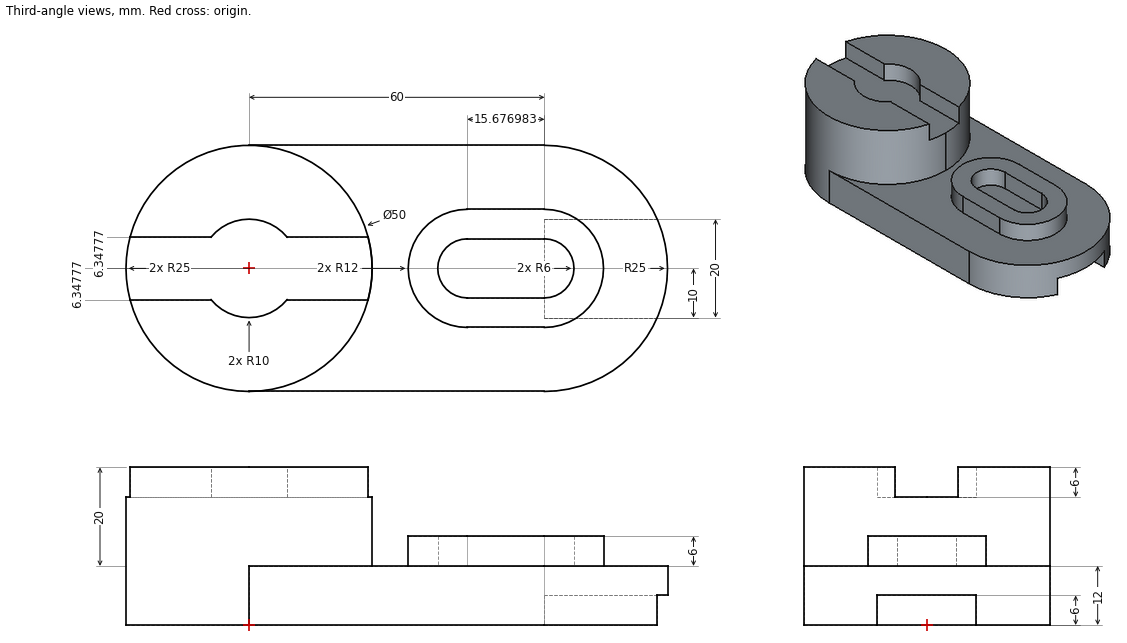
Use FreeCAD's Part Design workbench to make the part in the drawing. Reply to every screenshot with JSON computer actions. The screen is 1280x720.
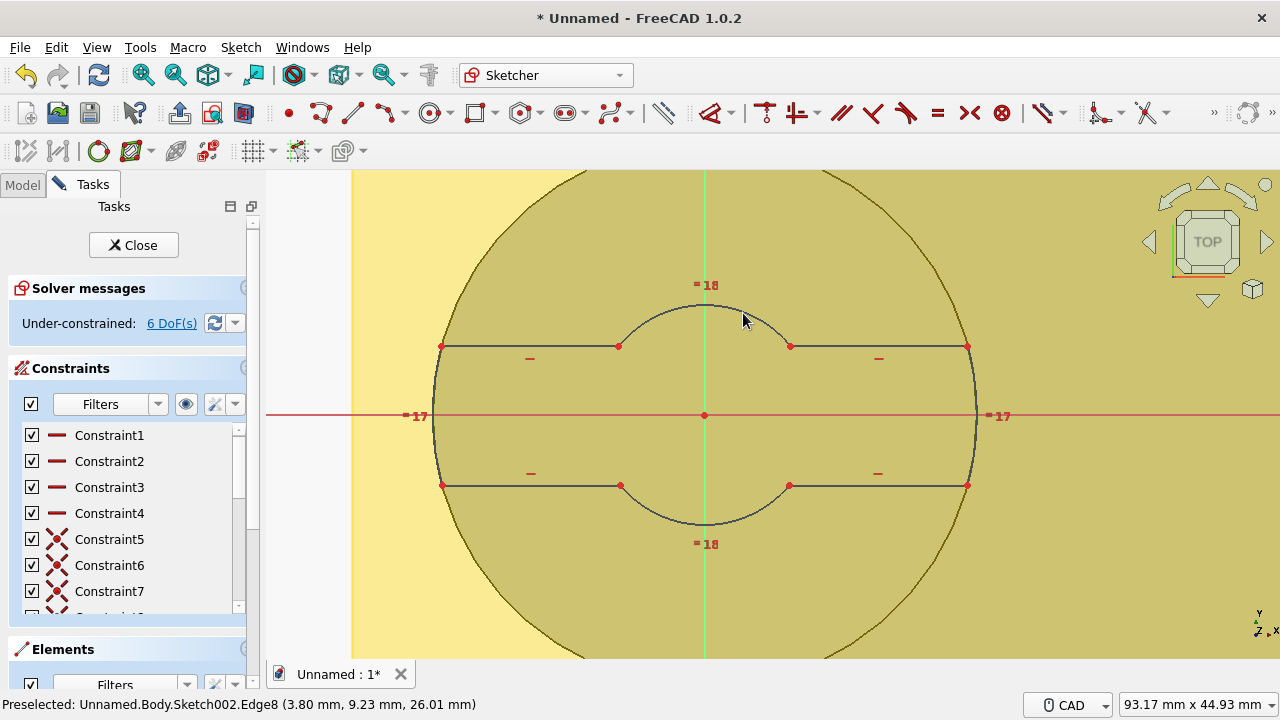
{"action": "left_click", "coordinate": [710, 114]}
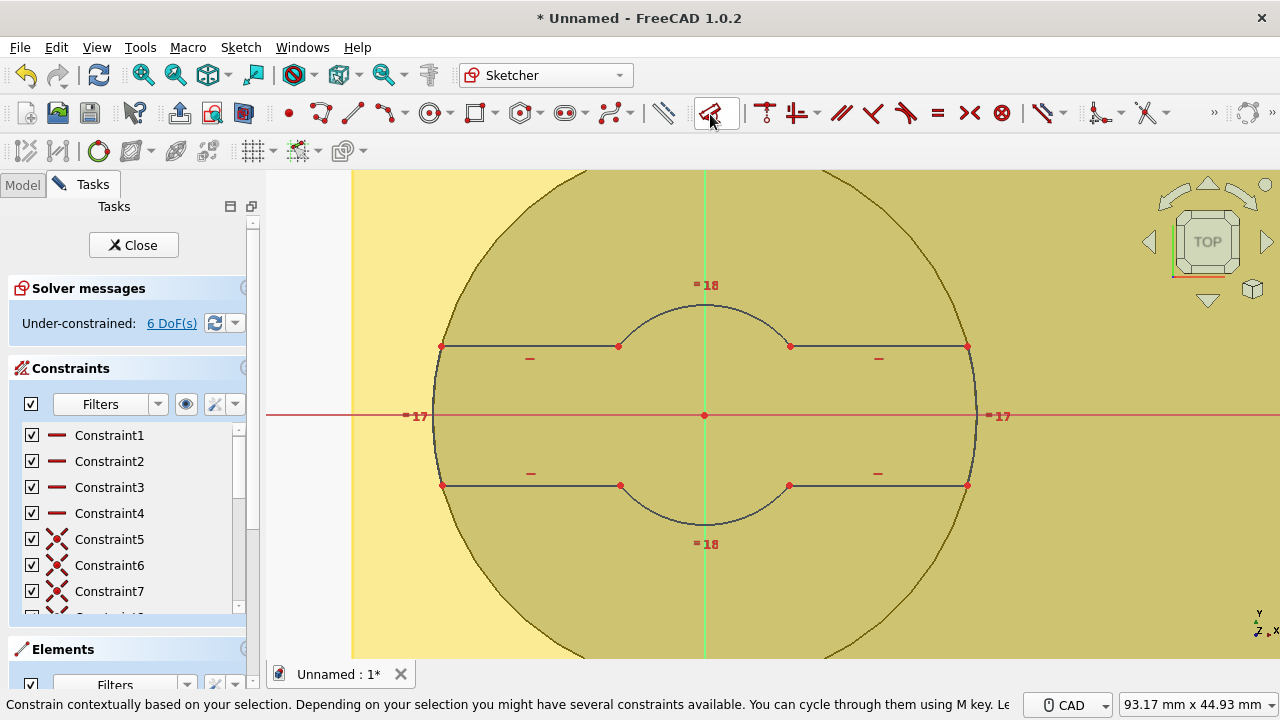
{"action": "left_click", "coordinate": [434, 388]}
{"action": "left_click", "coordinate": [402, 385]}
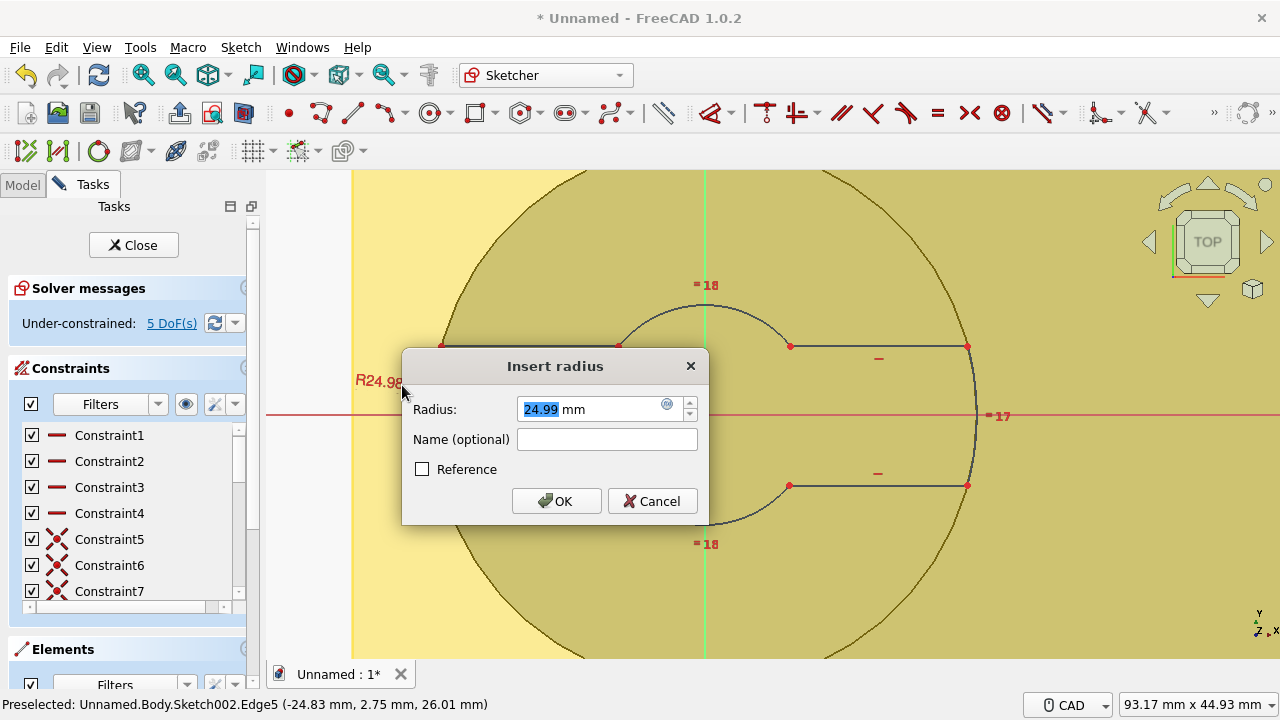
{"action": "type", "text": "25"}
{"action": "key", "text": "Return"}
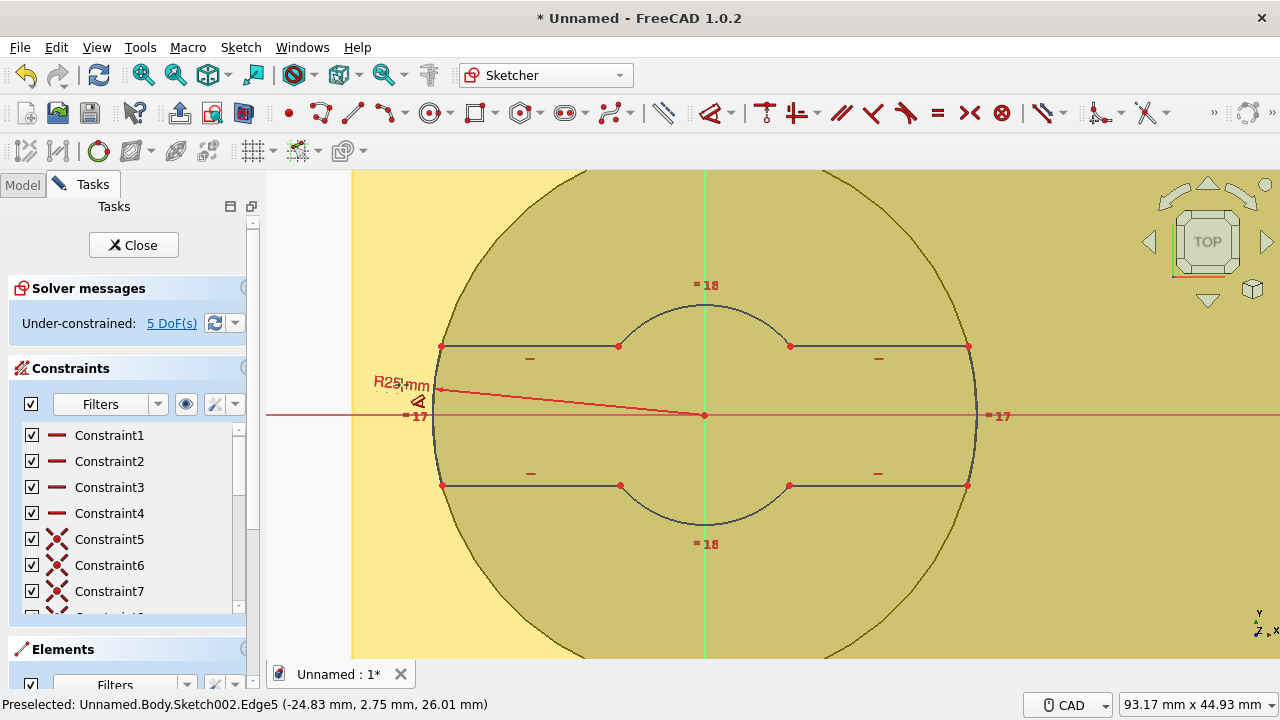
{"action": "left_click", "coordinate": [667, 518]}
{"action": "left_click", "coordinate": [656, 548]}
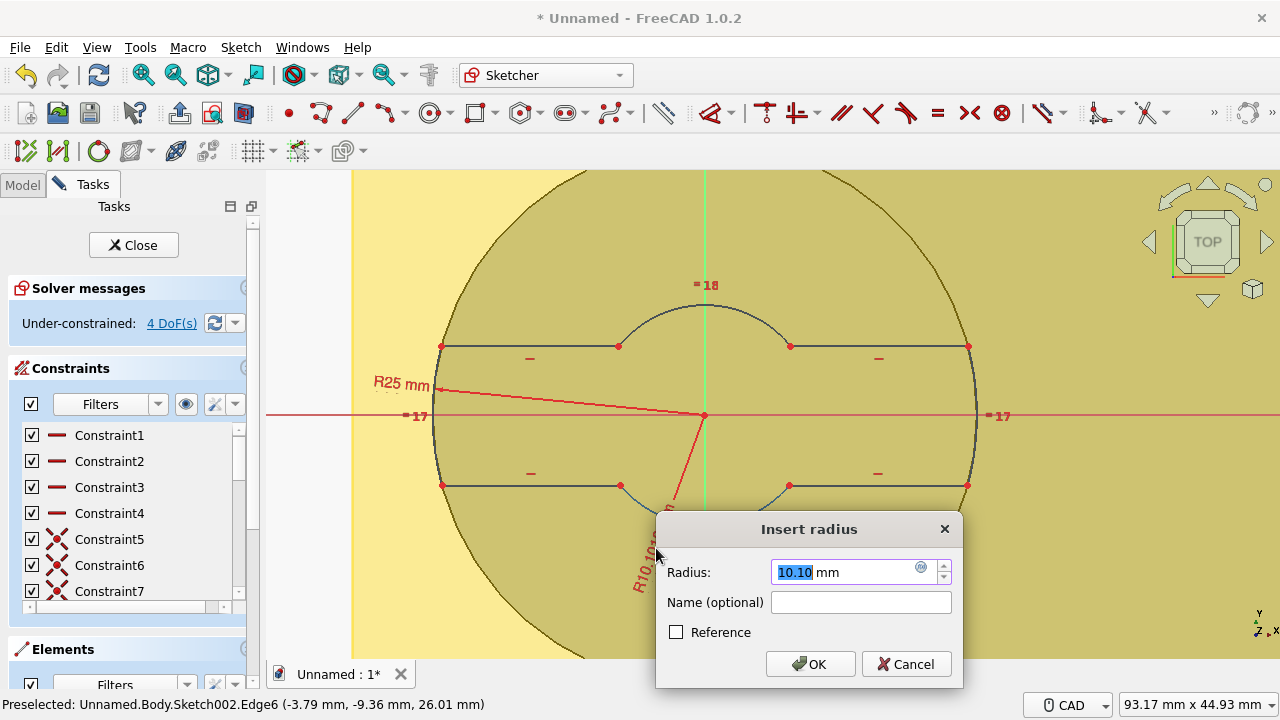
{"action": "type", "text": "10"}
{"action": "key", "text": "Return"}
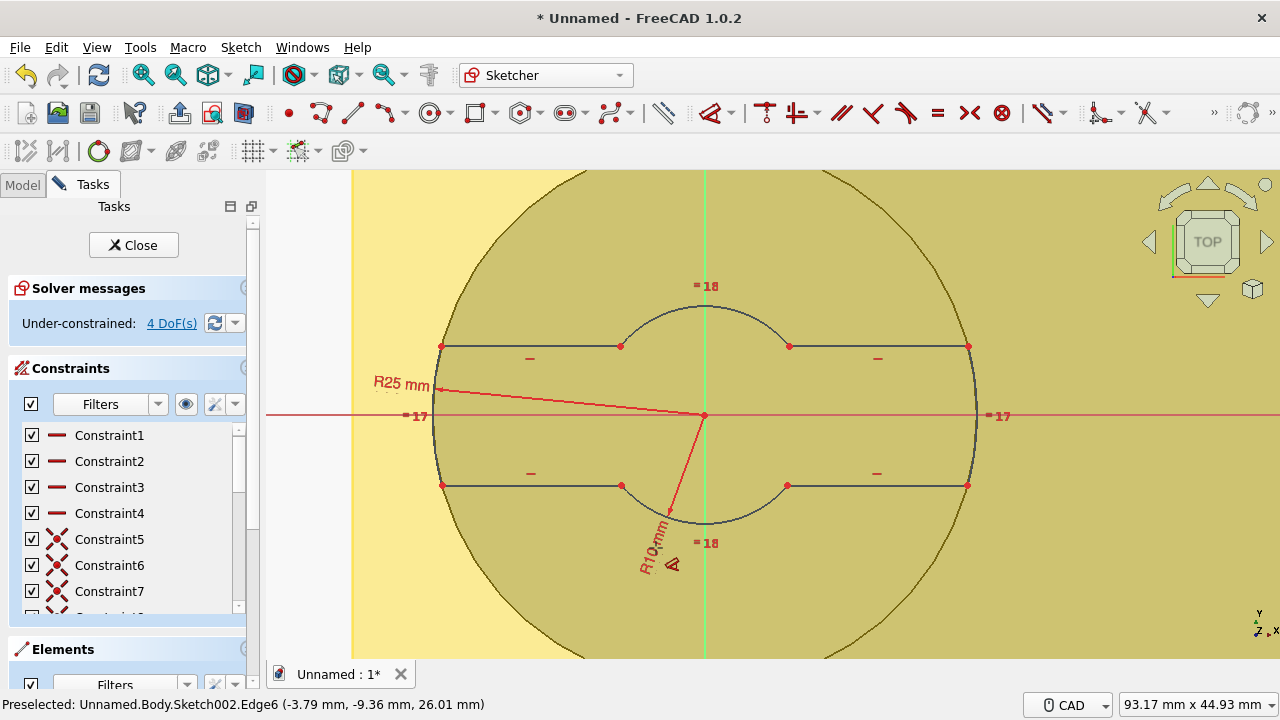
{"action": "left_click", "coordinate": [620, 346]}
{"action": "left_click", "coordinate": [586, 381]}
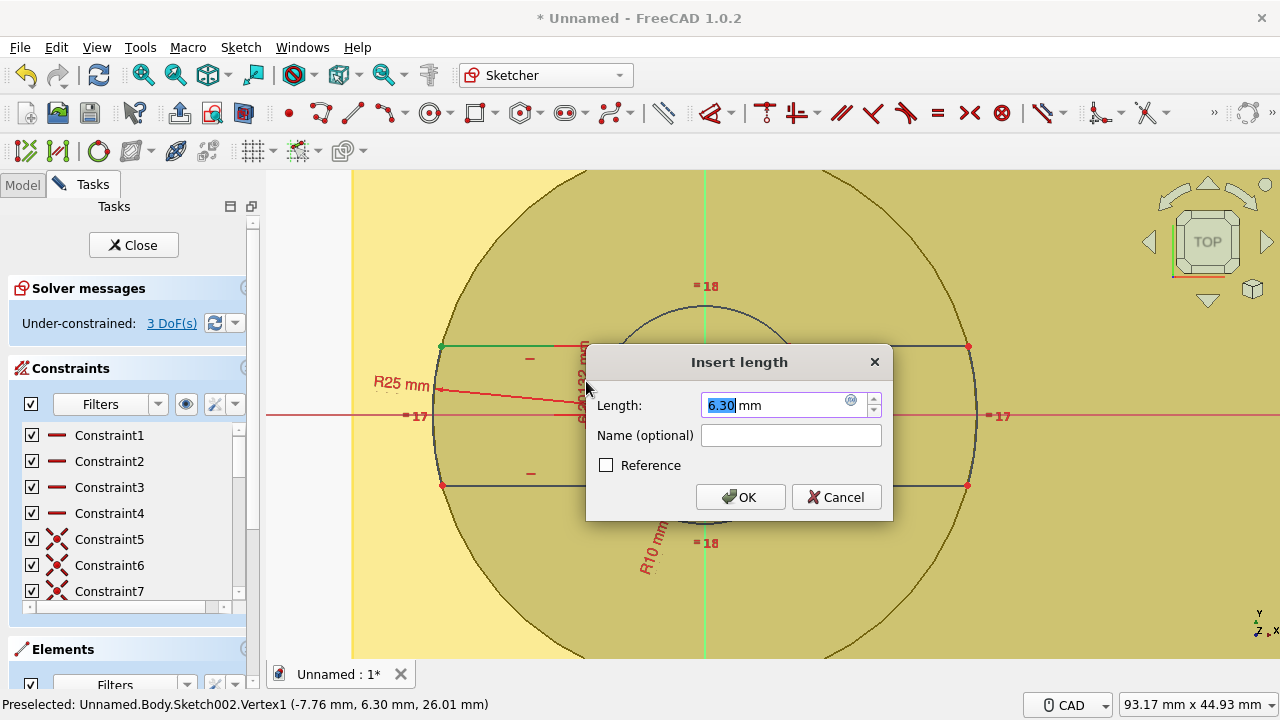
{"action": "type", "text": "6.34777"}
{"action": "key", "text": "Return"}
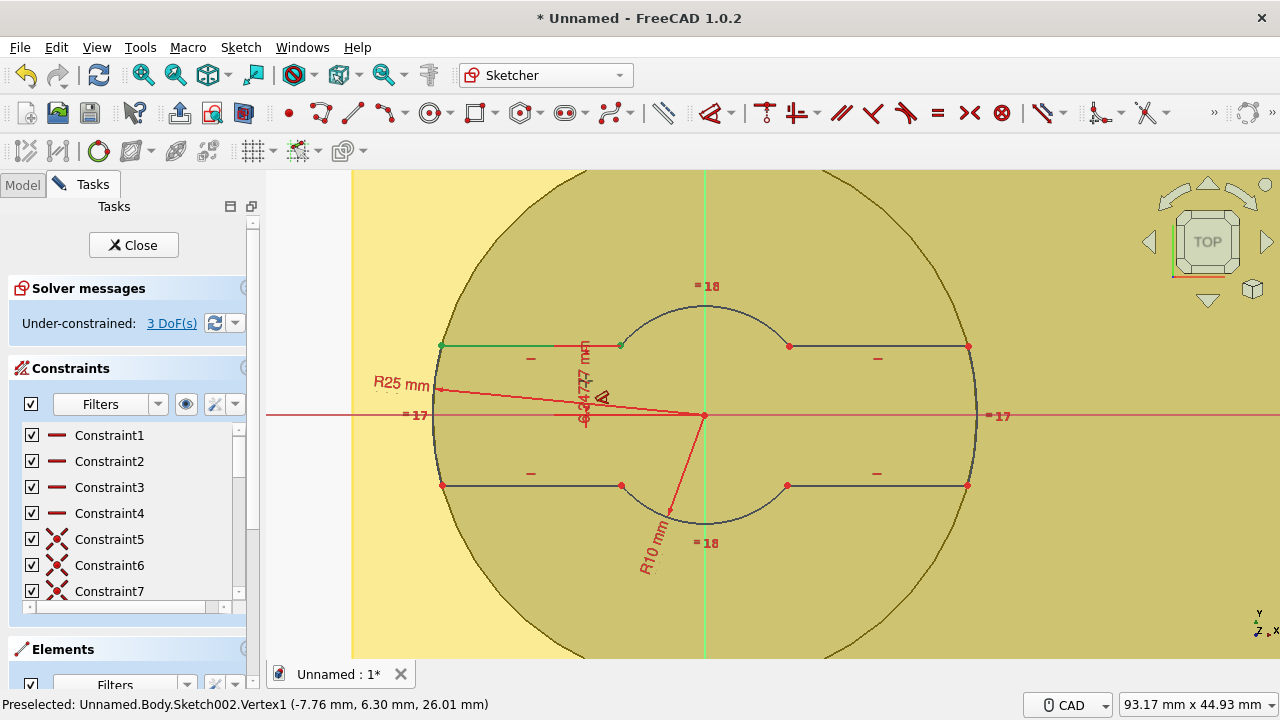
{"action": "left_click", "coordinate": [442, 486]}
{"action": "left_click", "coordinate": [408, 450]}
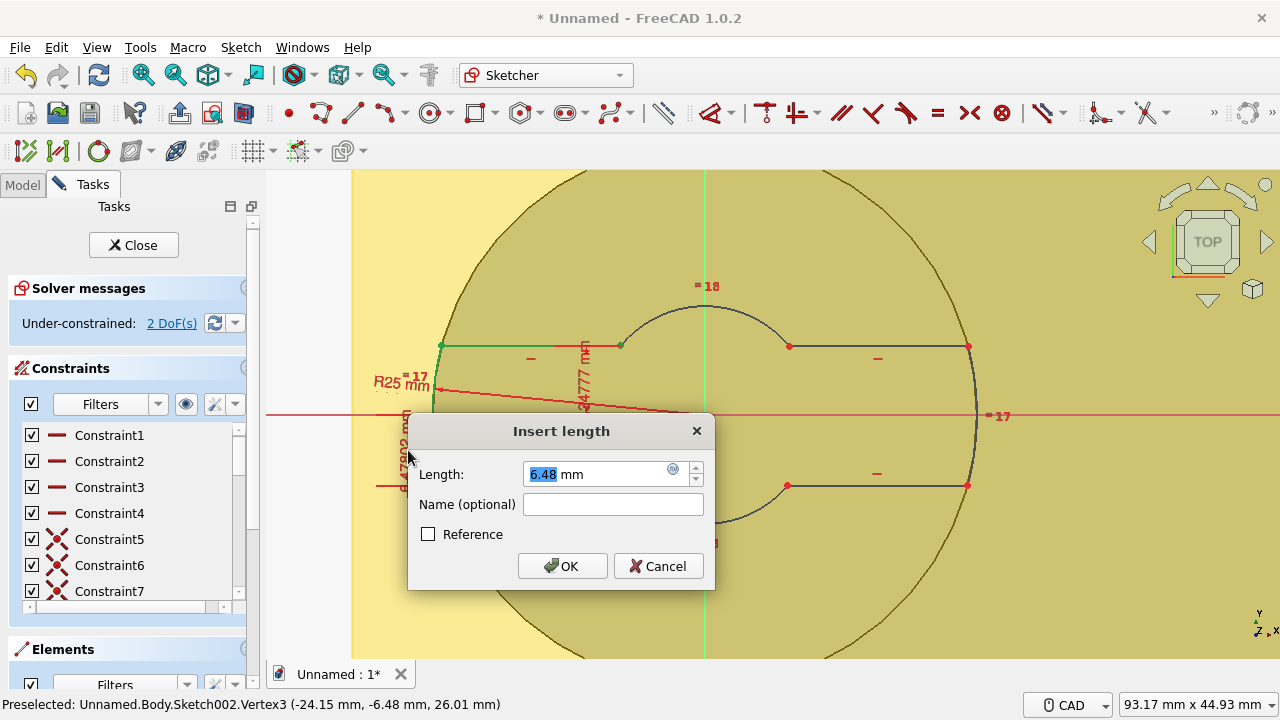
{"action": "type", "text": "6.34777"}
{"action": "key", "text": "Return"}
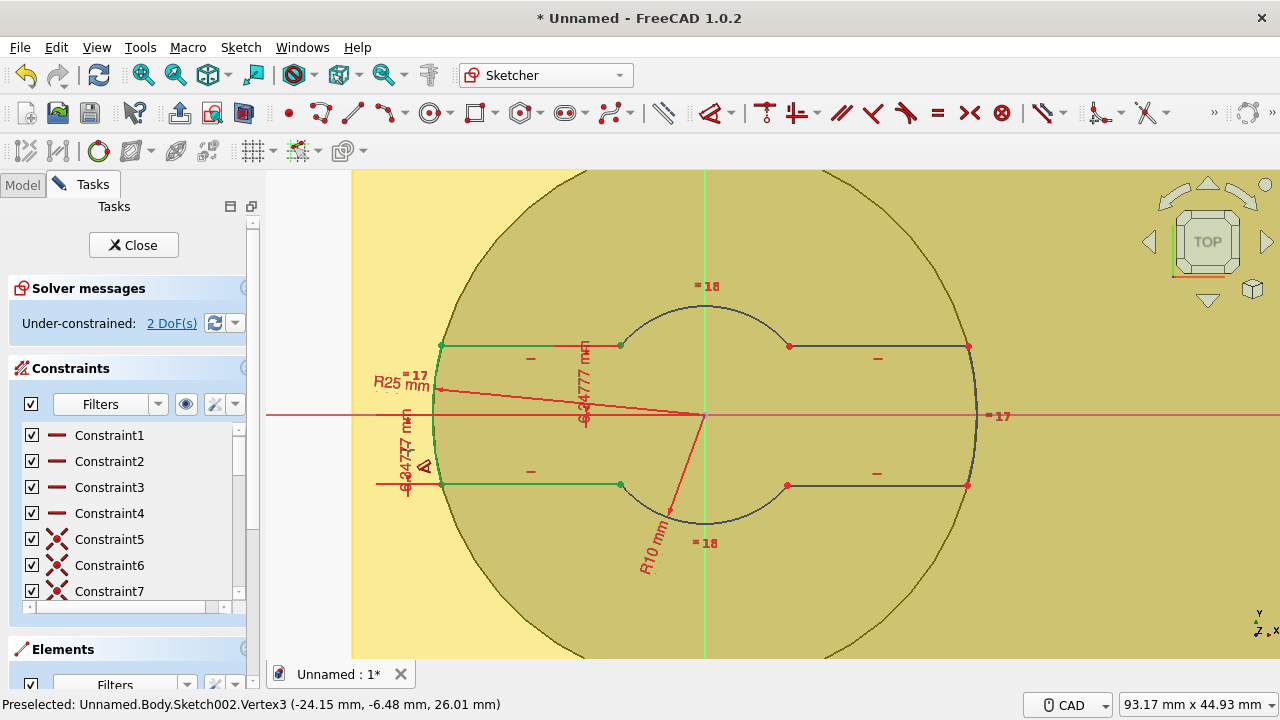
{"action": "left_click", "coordinate": [788, 486]}
{"action": "left_click", "coordinate": [822, 450]}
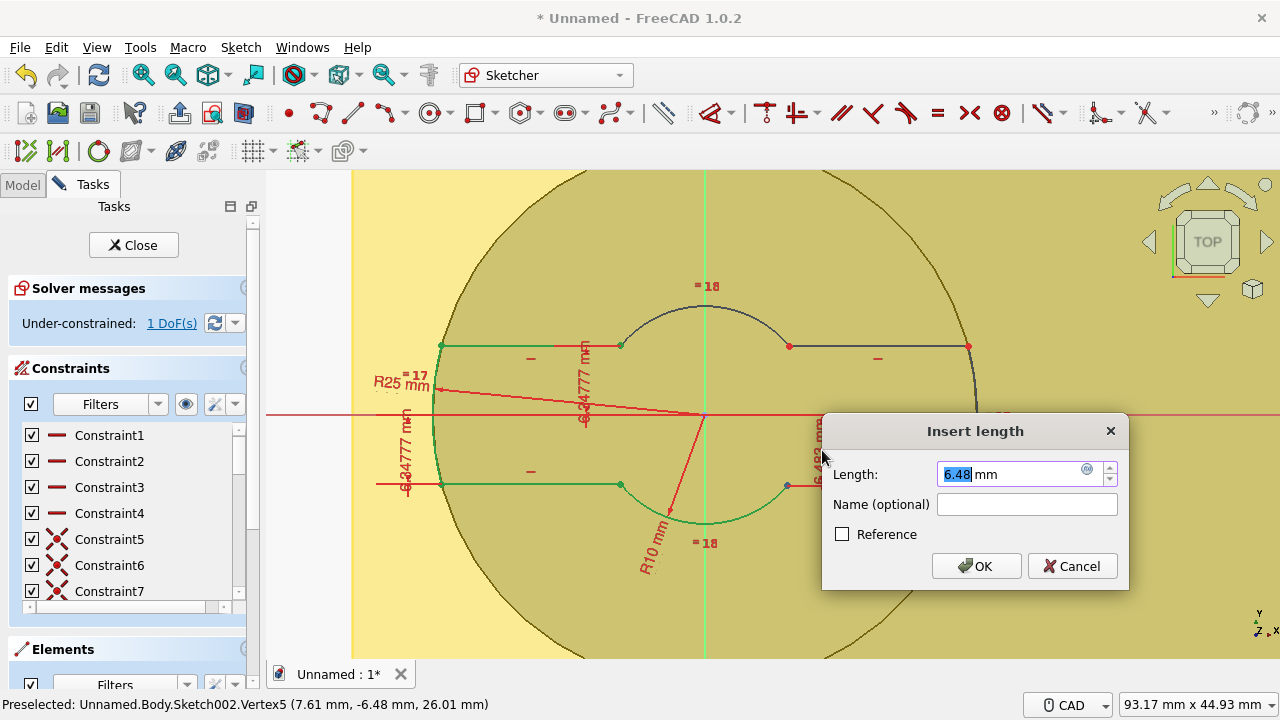
{"action": "type", "text": "6.34777"}
{"action": "key", "text": "Return"}